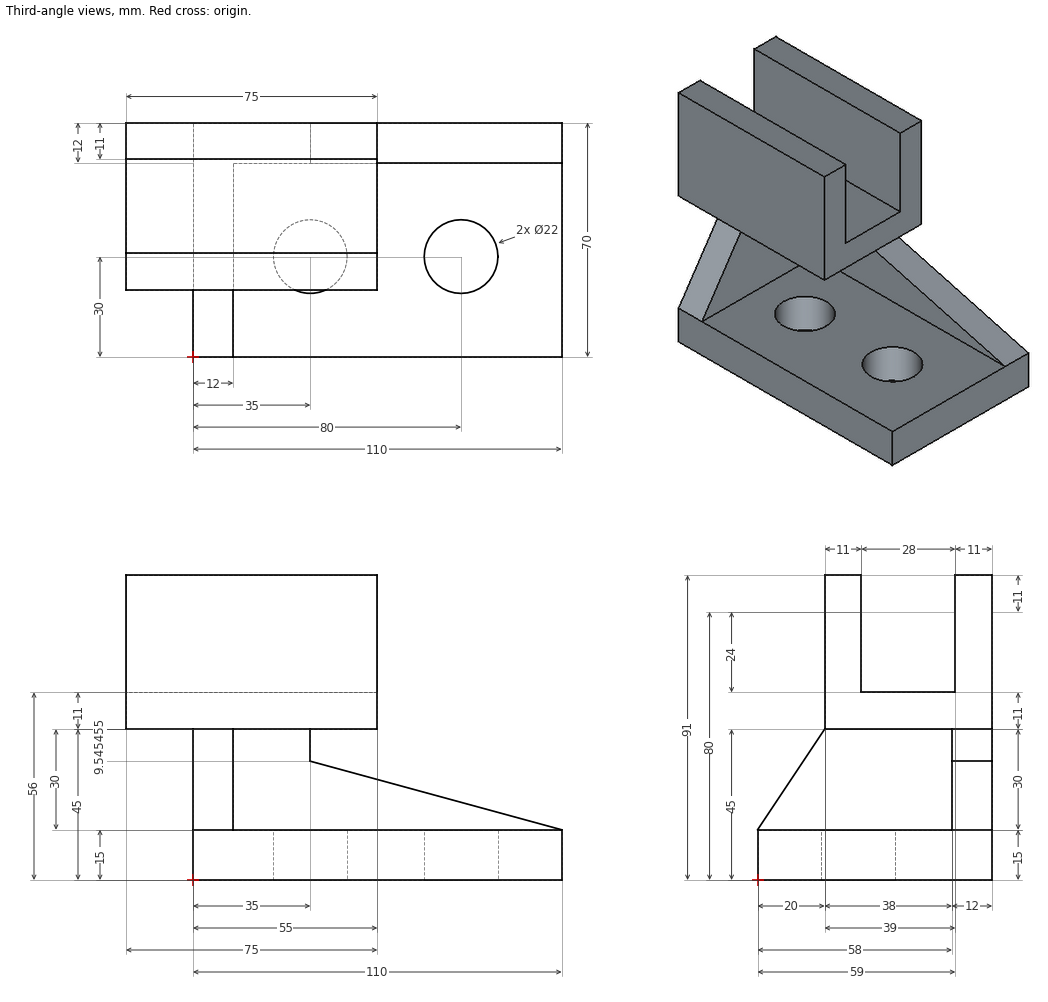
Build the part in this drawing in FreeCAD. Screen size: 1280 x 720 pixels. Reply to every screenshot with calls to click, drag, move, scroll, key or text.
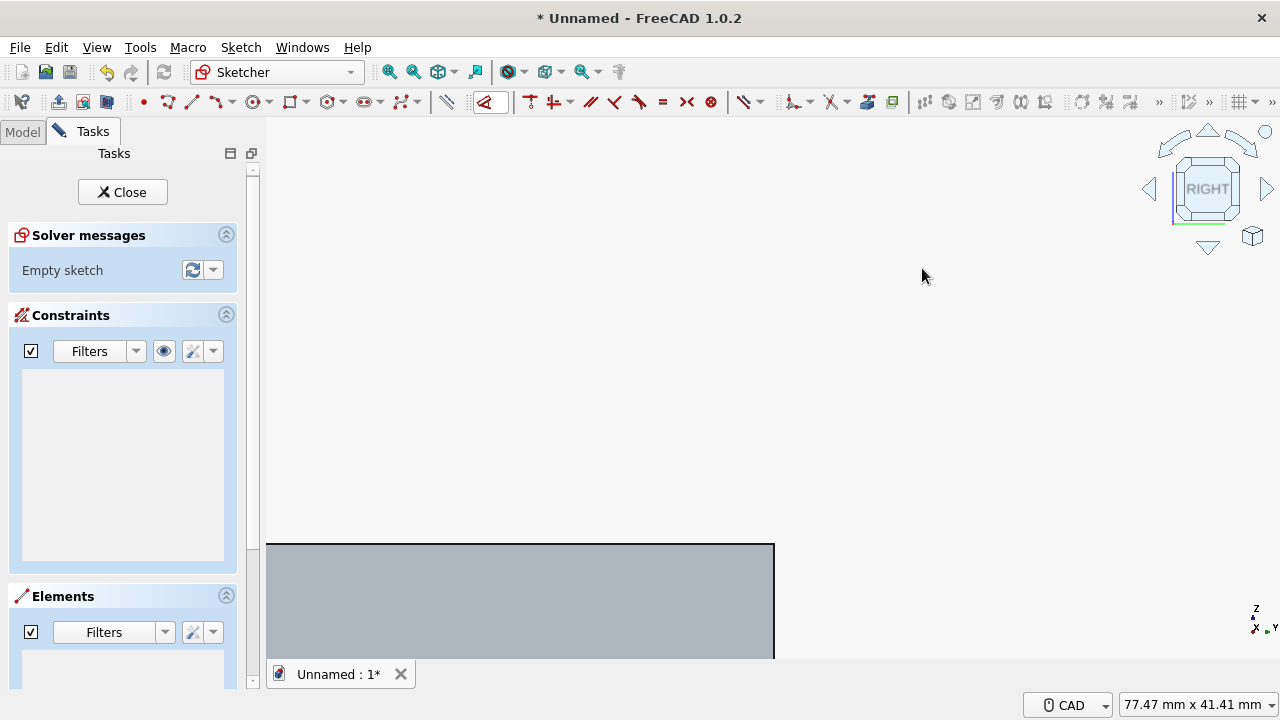
click(290, 102)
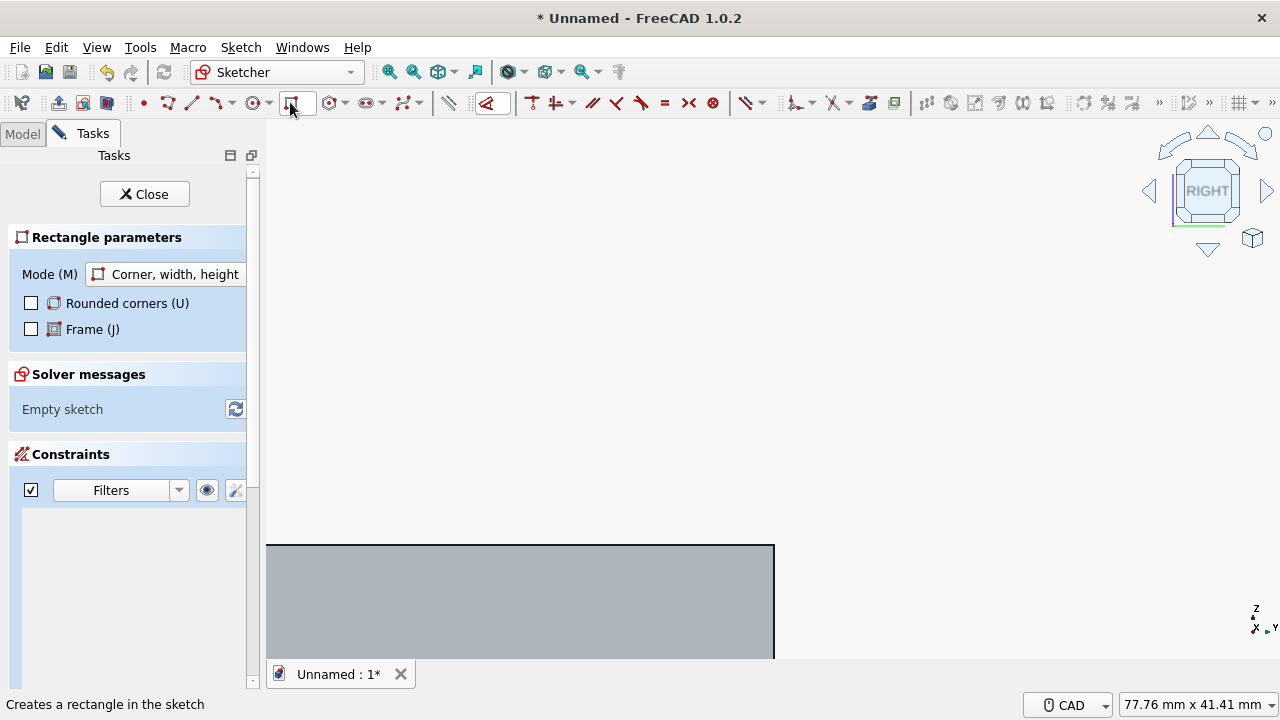
click(630, 232)
move(774, 545)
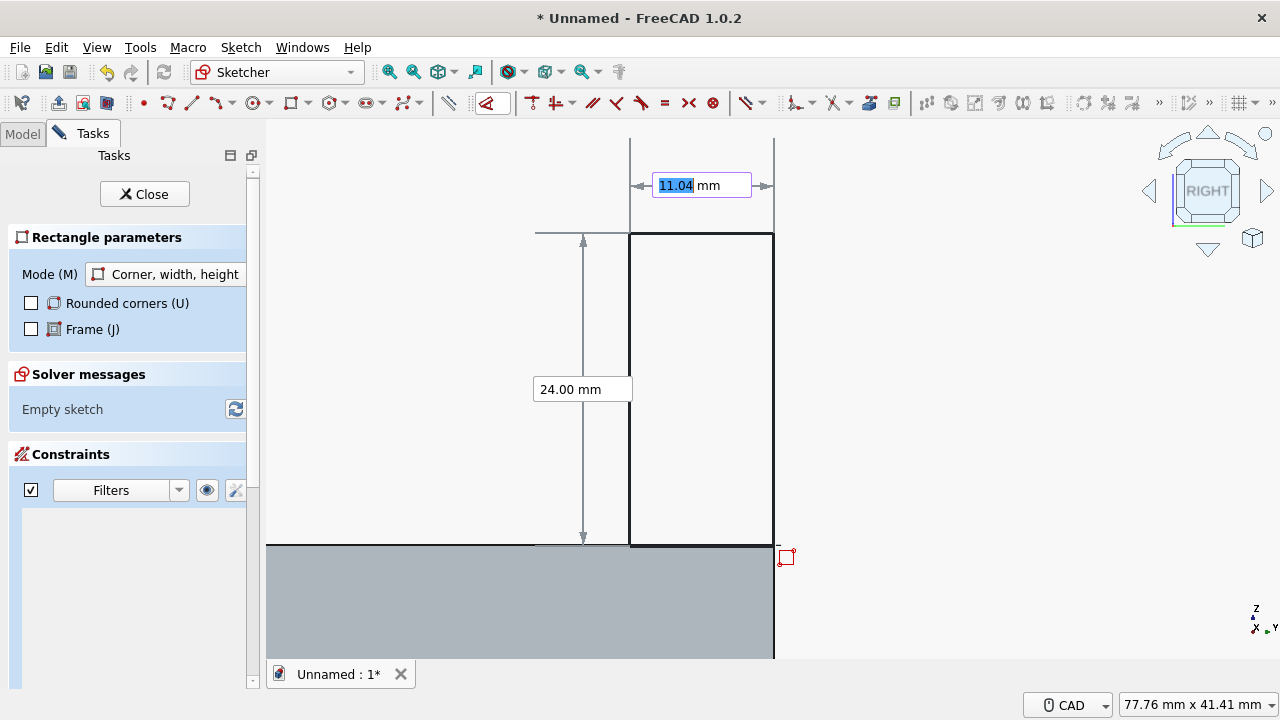
text(11)
key(Tab)
text(24)
key(Return)
key(Escape)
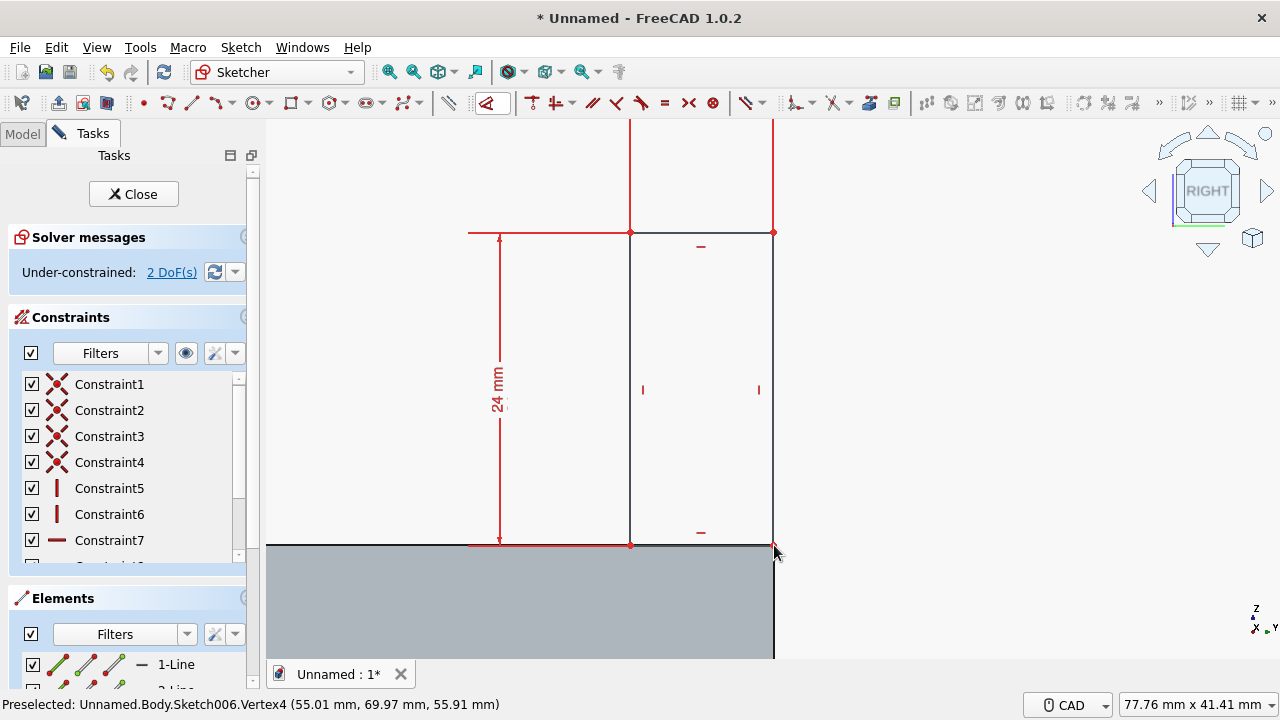
click(630, 233)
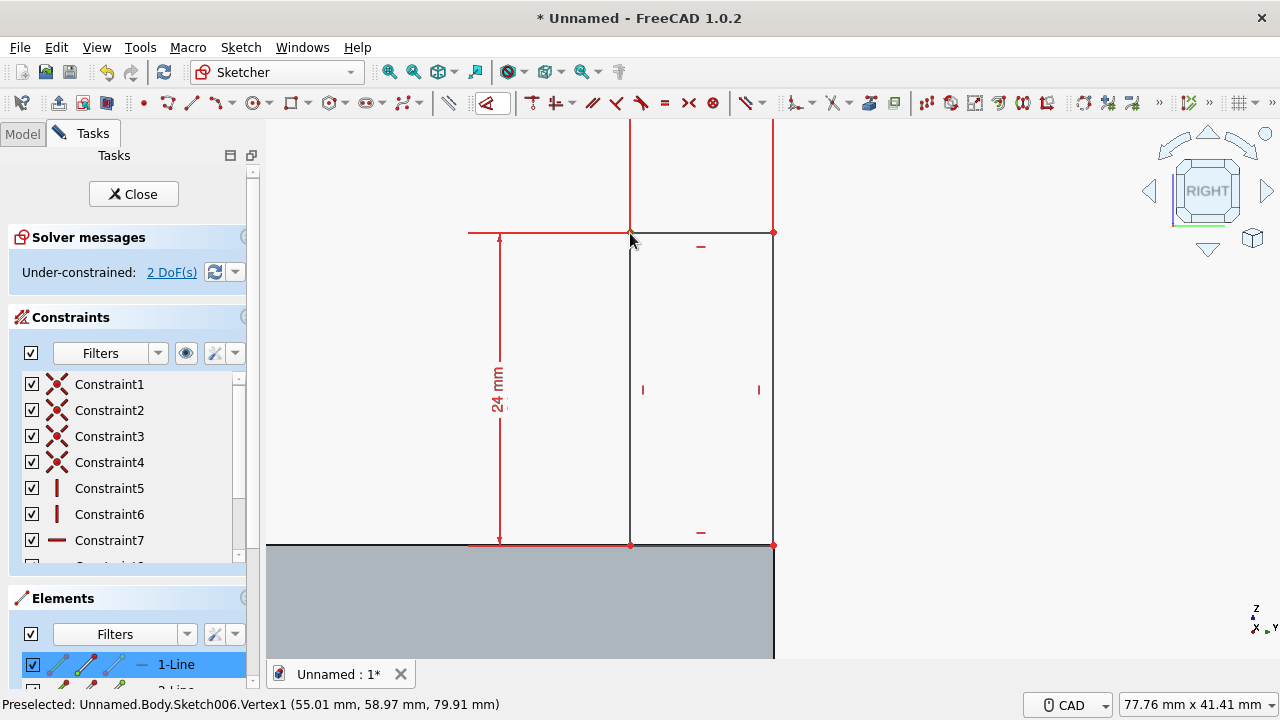
click(504, 104)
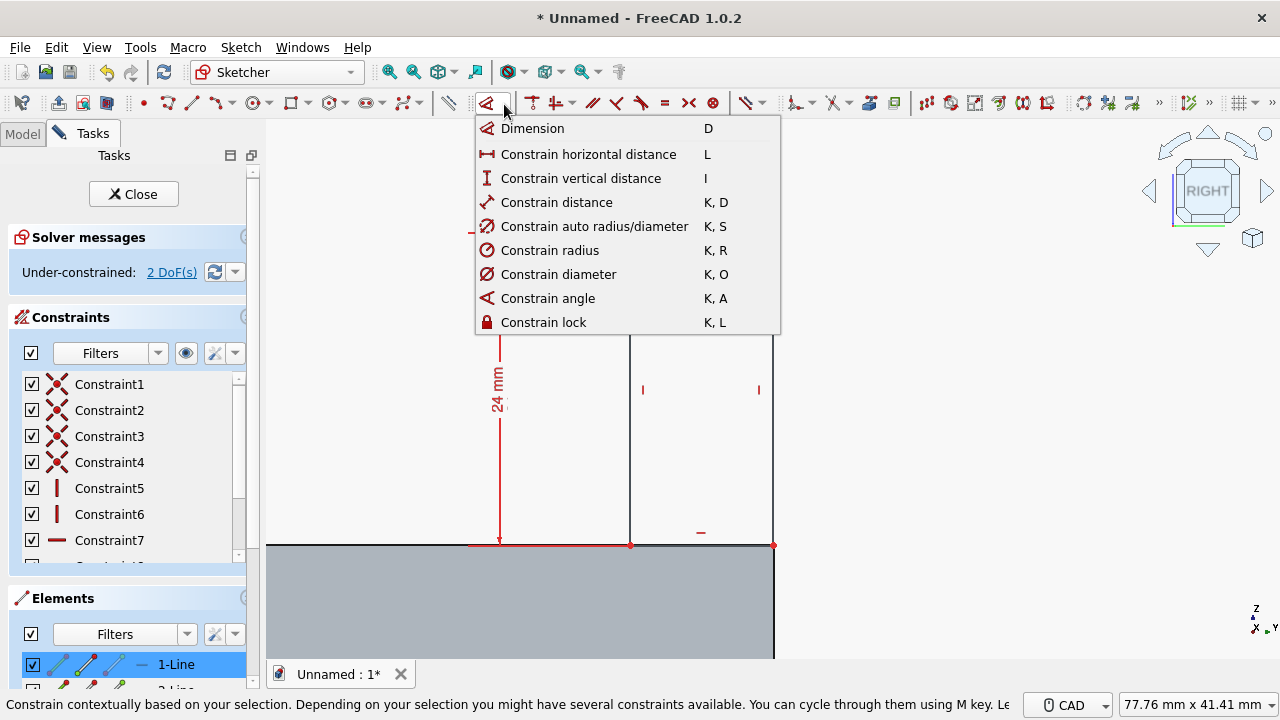
click(628, 154)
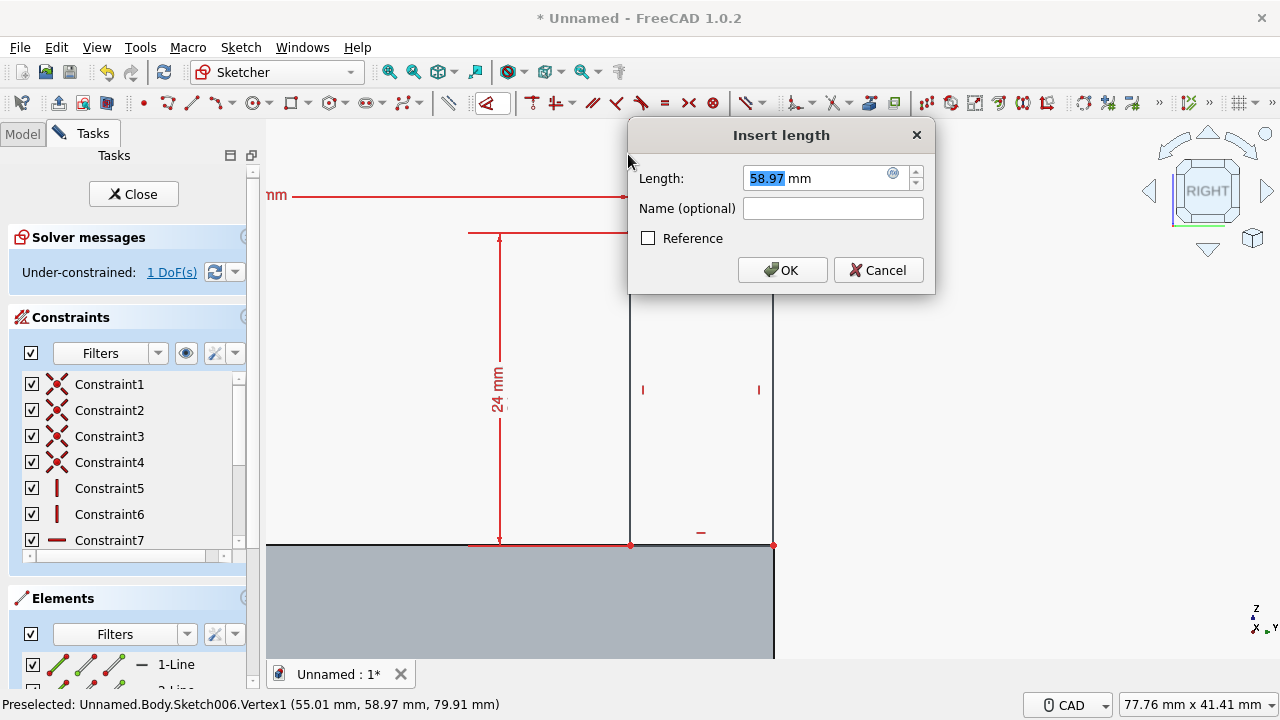
text(59)
key(Return)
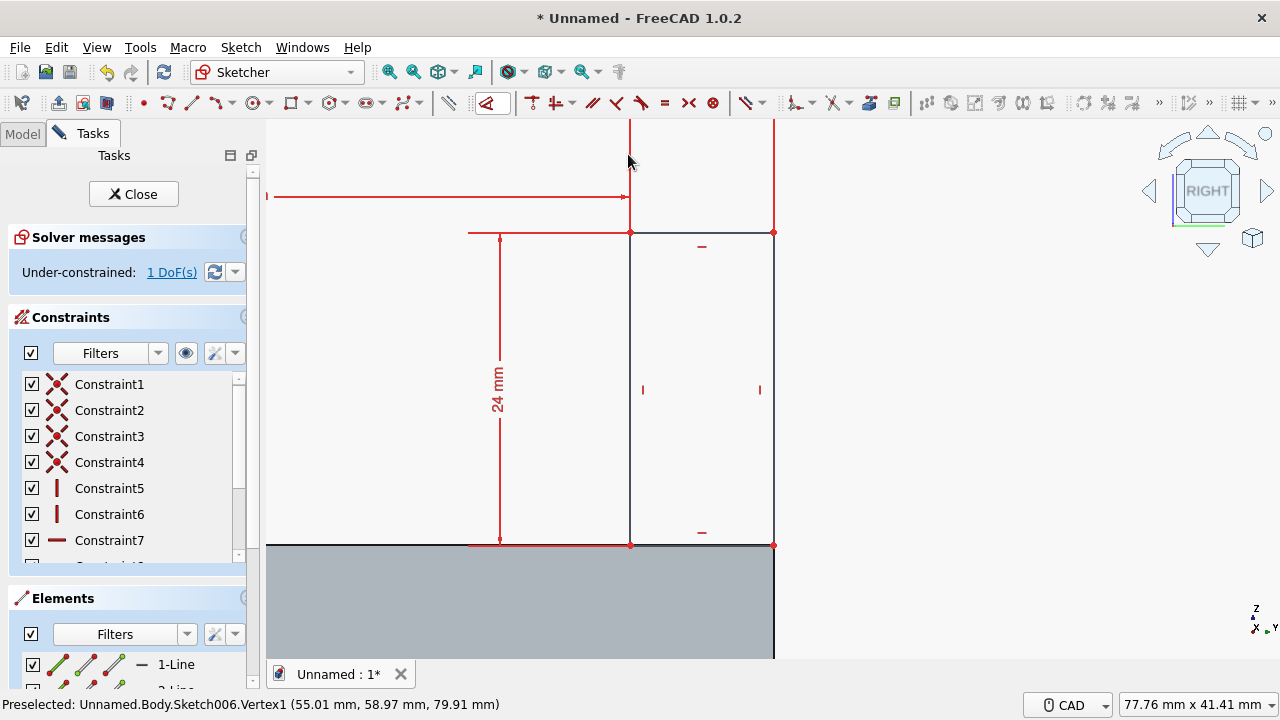
click(630, 233)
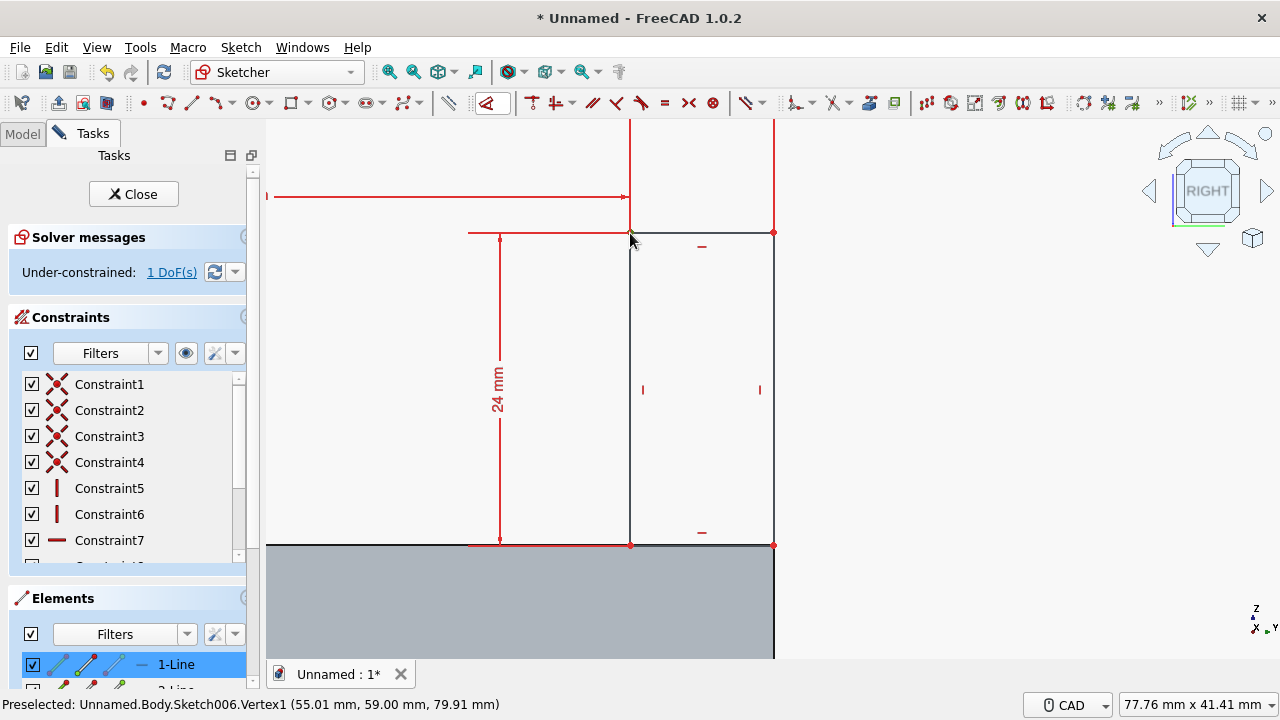
click(504, 104)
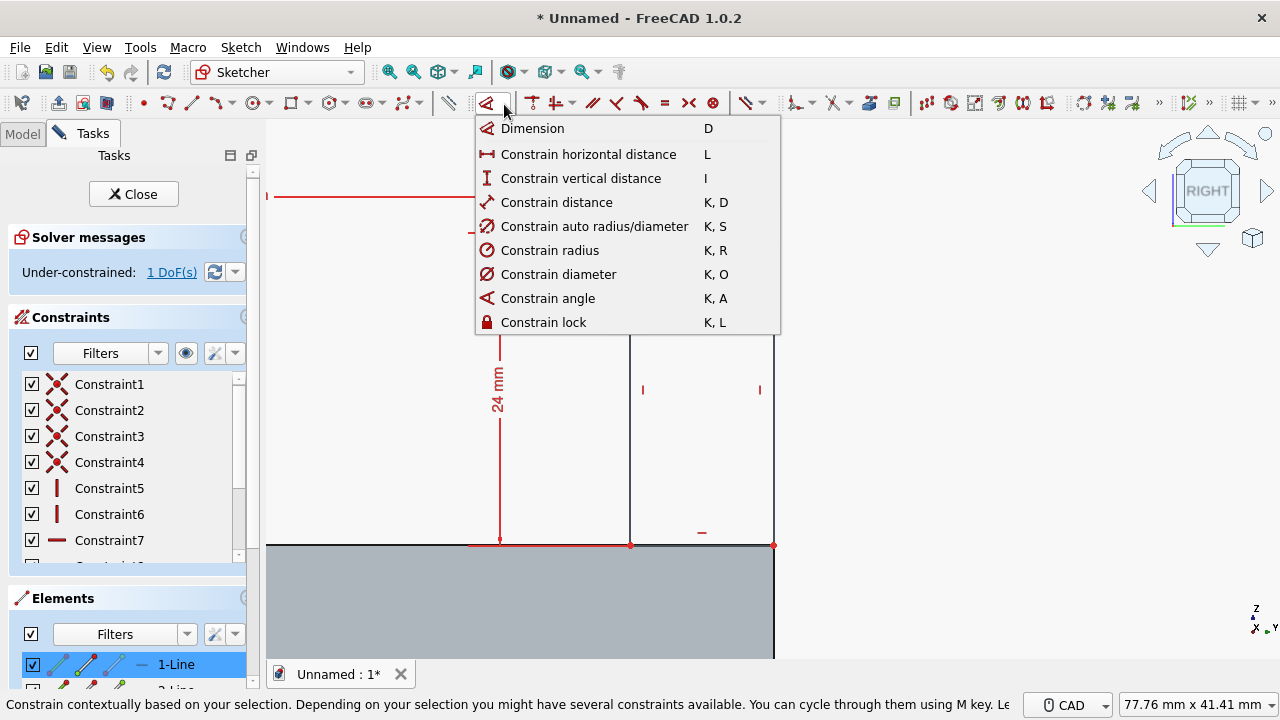
click(628, 178)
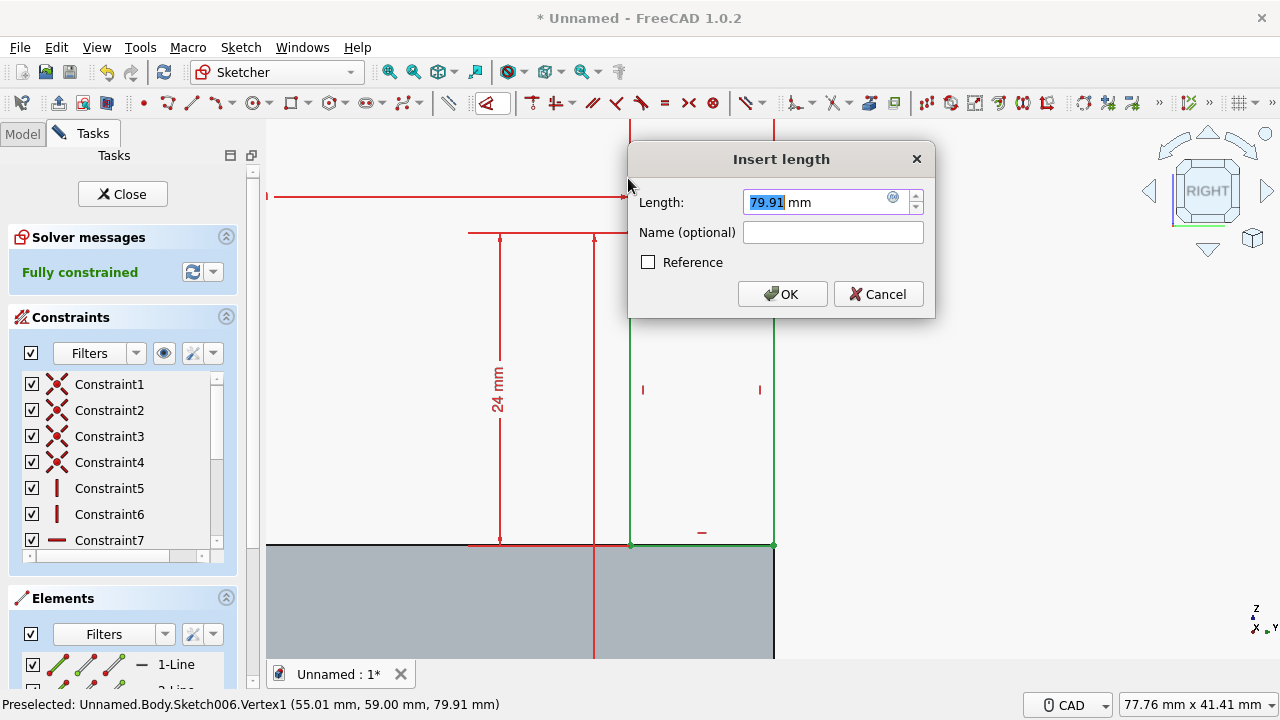
text(80)
key(Return)